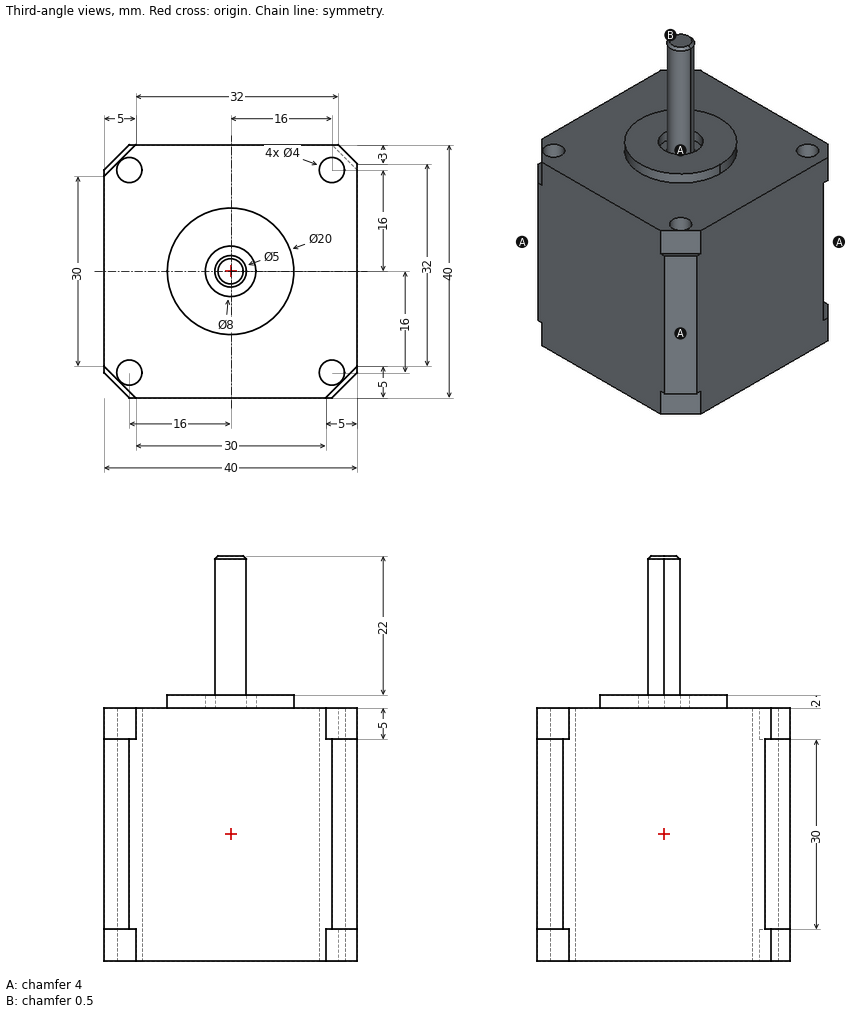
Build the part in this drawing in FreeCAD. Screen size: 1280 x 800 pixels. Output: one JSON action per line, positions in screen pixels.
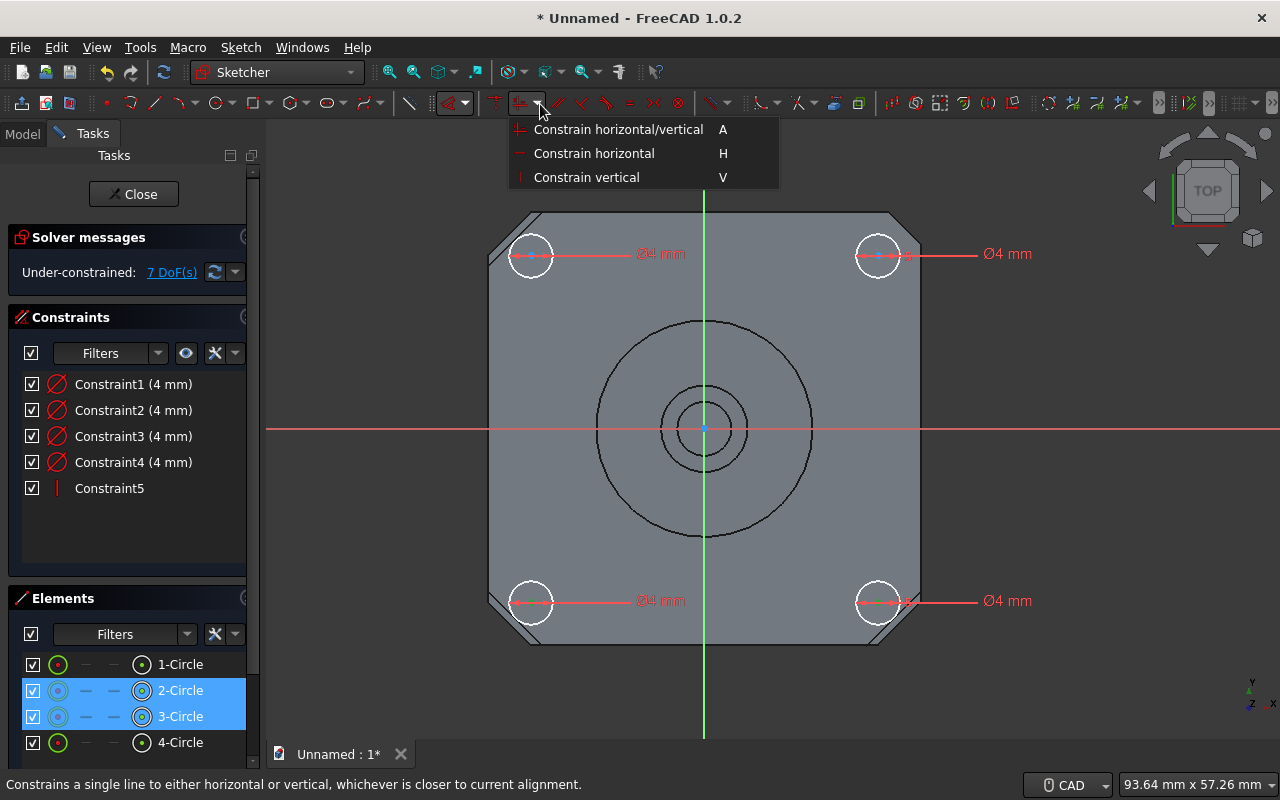
{"action": "left_click", "coordinate": [644, 153]}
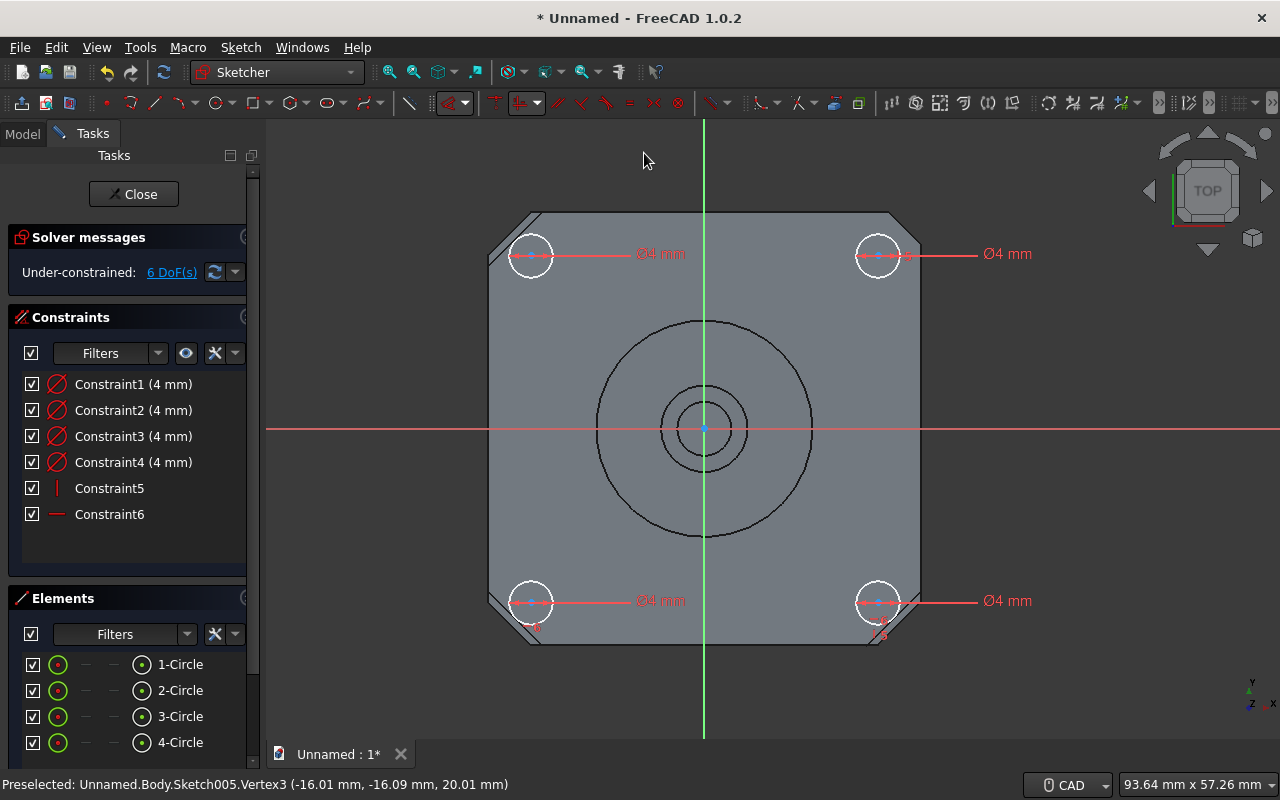
{"action": "left_click", "coordinate": [531, 603]}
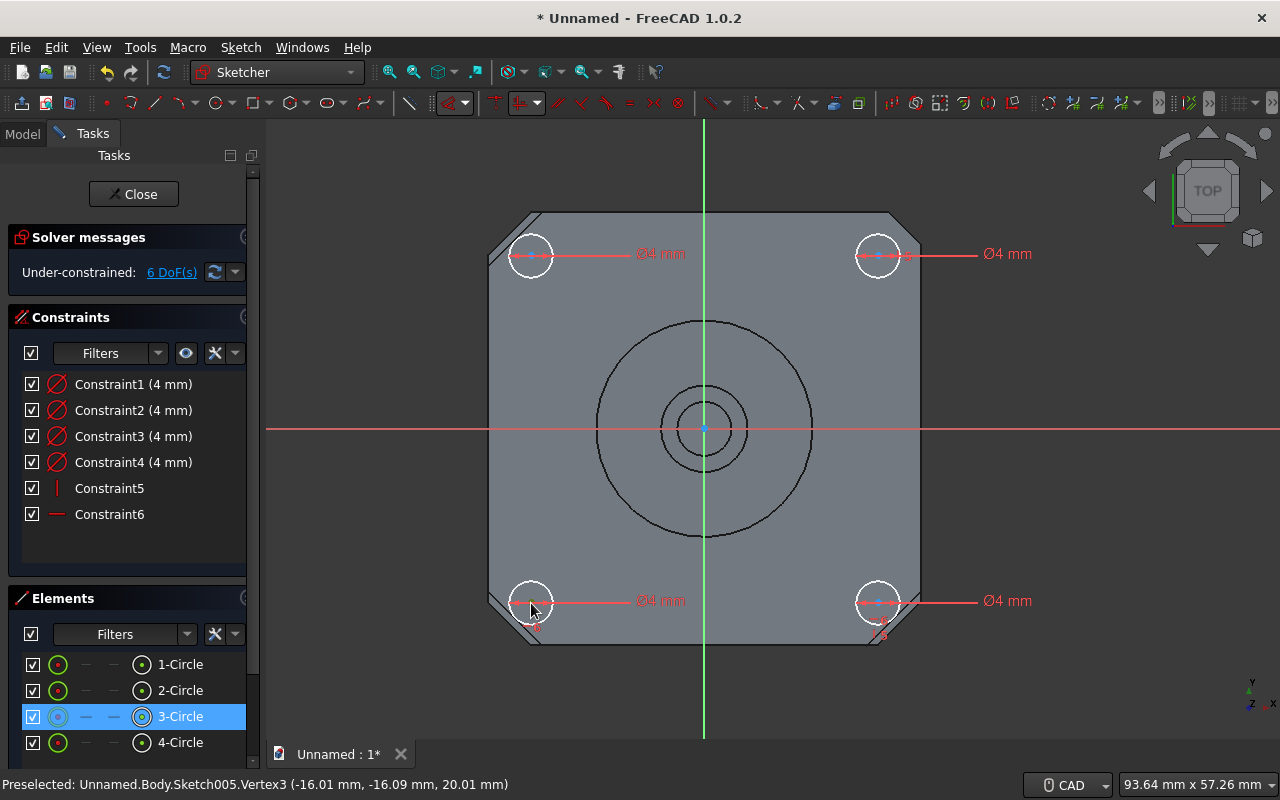
{"action": "left_click", "coordinate": [531, 256]}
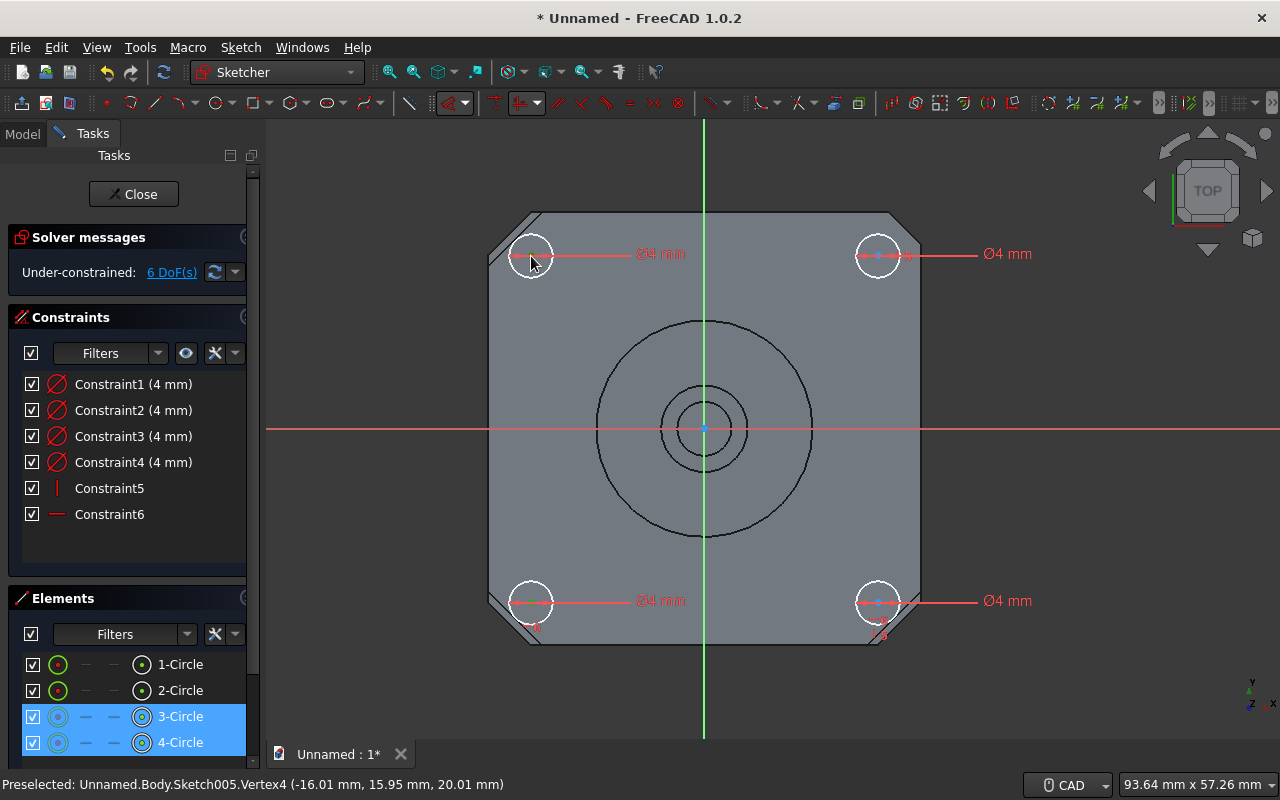
{"action": "key", "text": "v"}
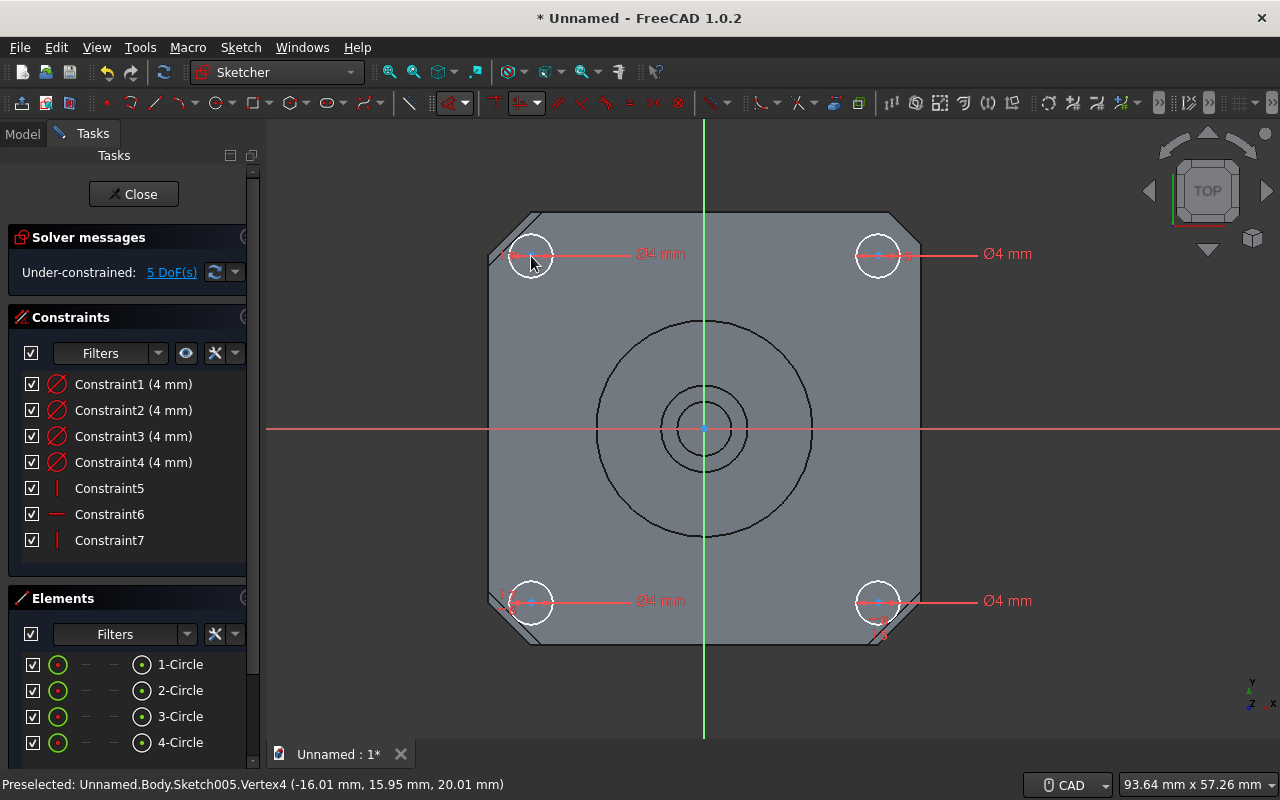
{"action": "left_click", "coordinate": [878, 256]}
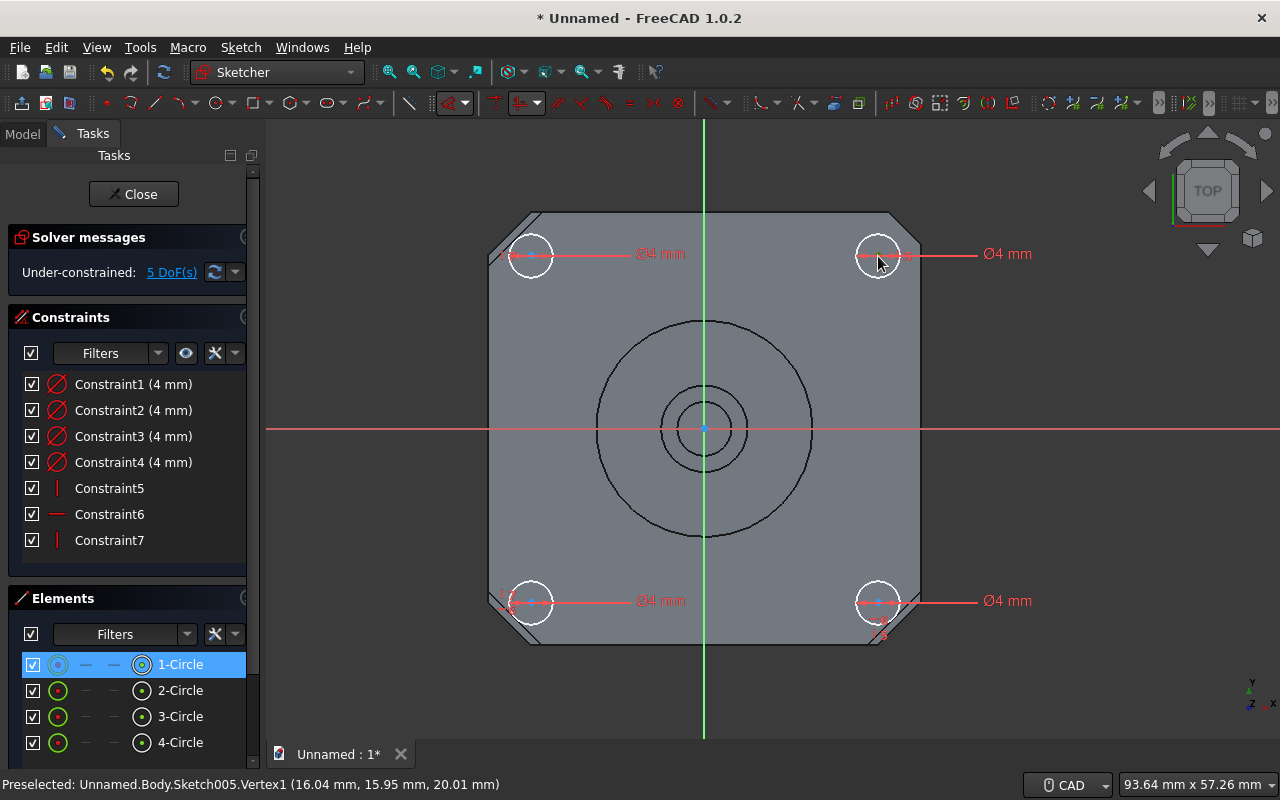
{"action": "left_click", "coordinate": [531, 256]}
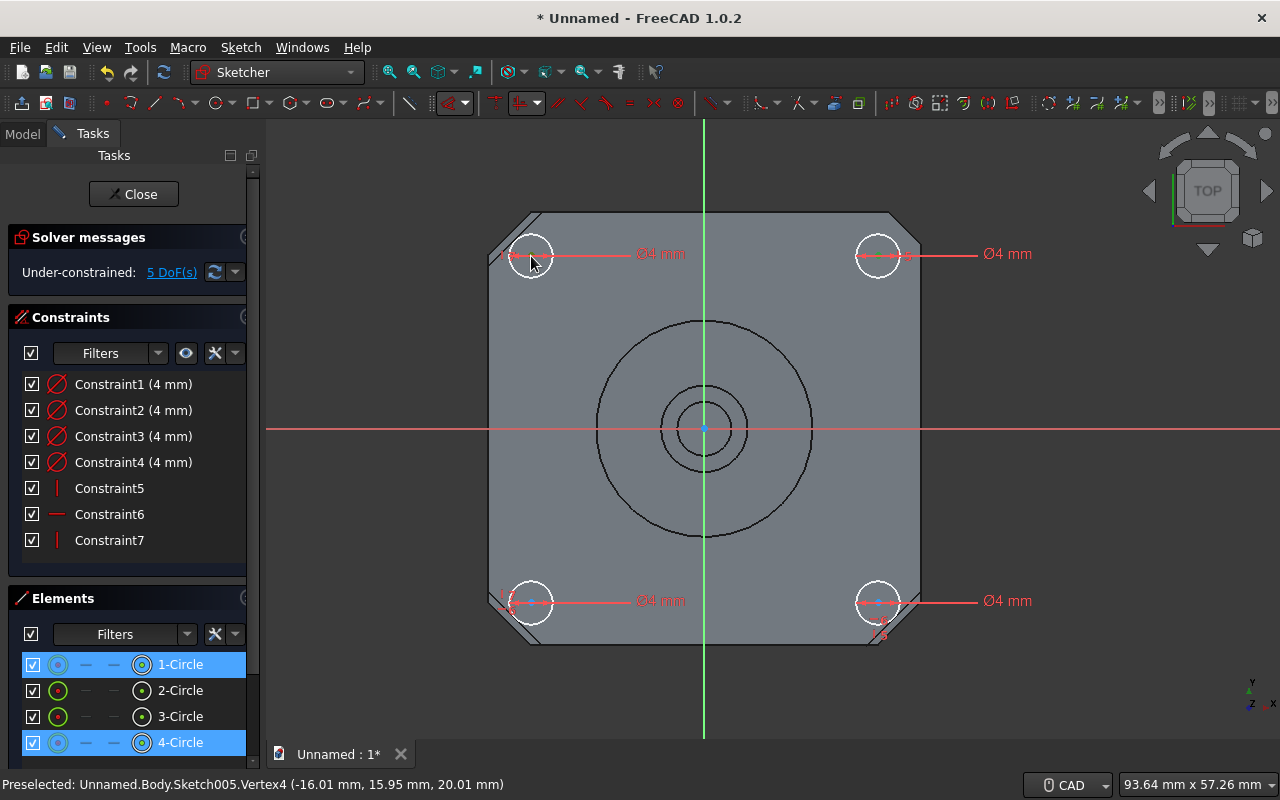
{"action": "left_click", "coordinate": [540, 104]}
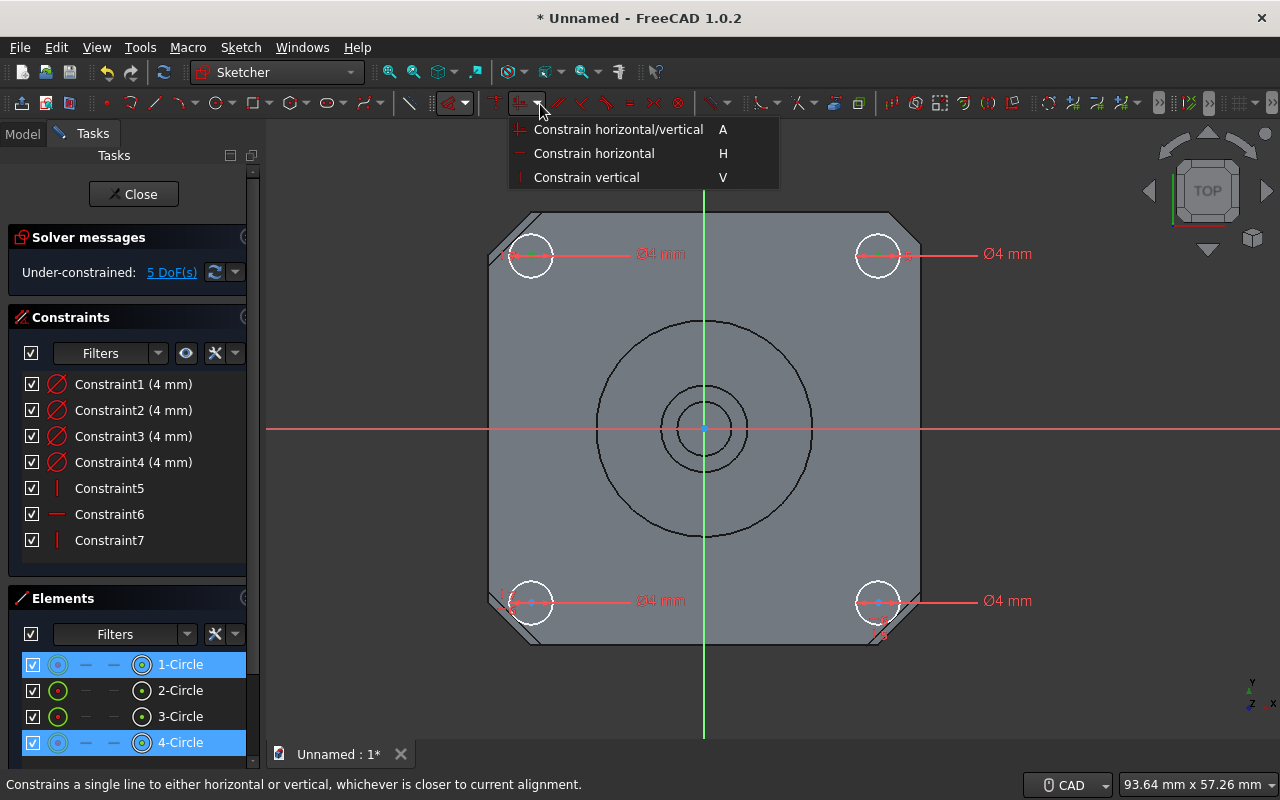
{"action": "left_click", "coordinate": [644, 153]}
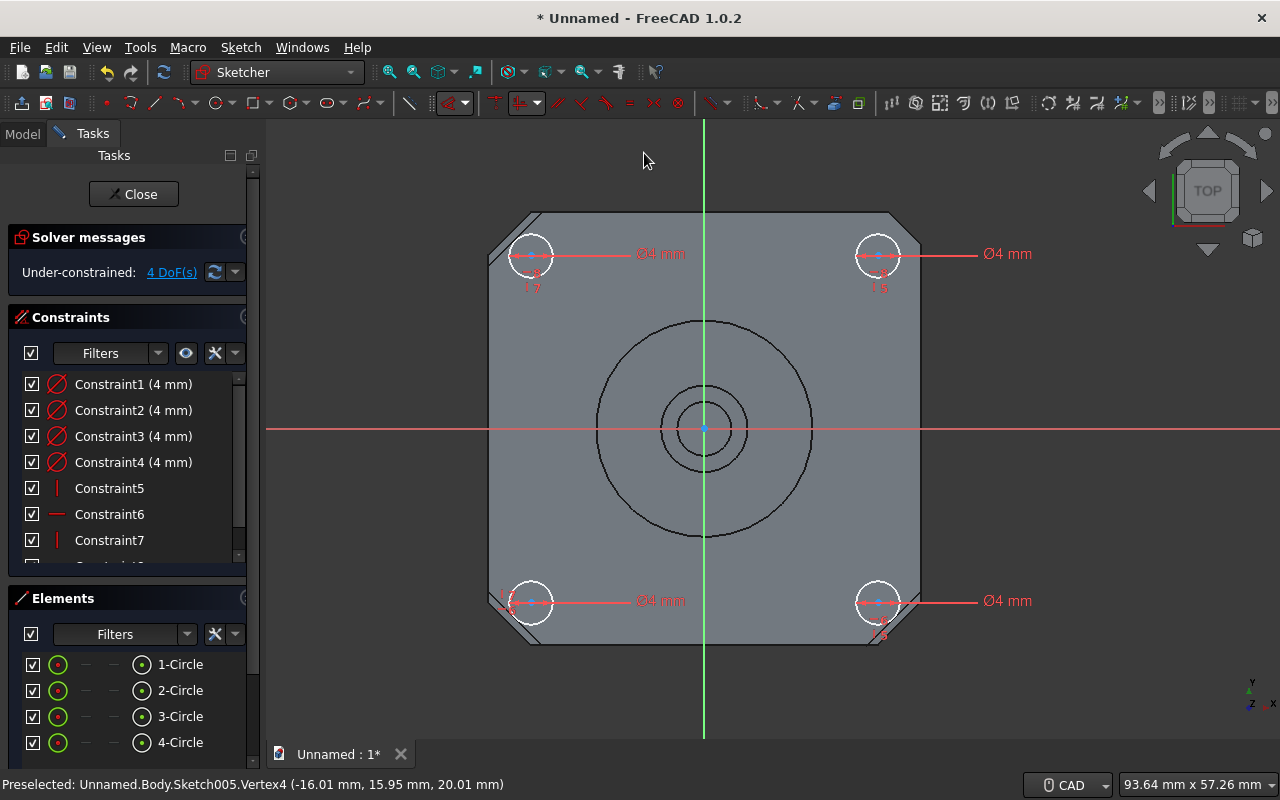
{"action": "left_click", "coordinate": [878, 256]}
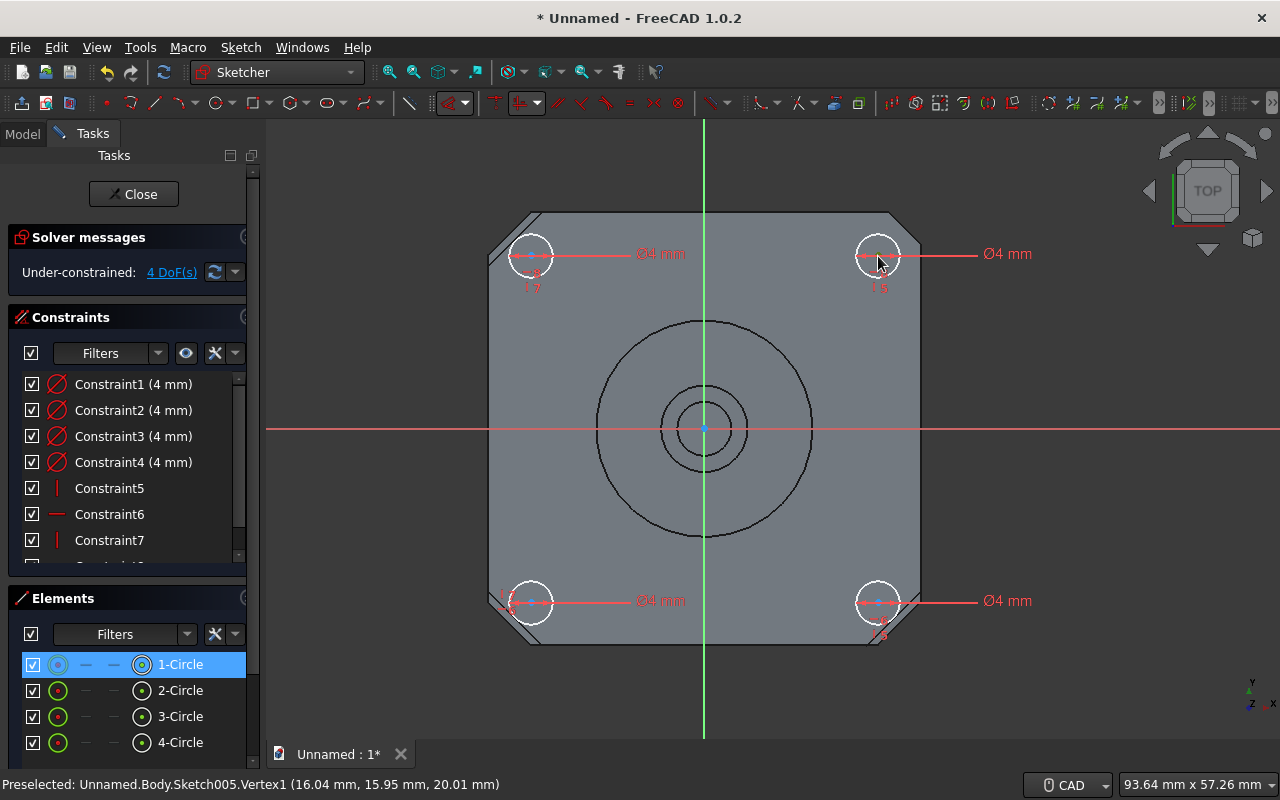
{"action": "key", "text": "l"}